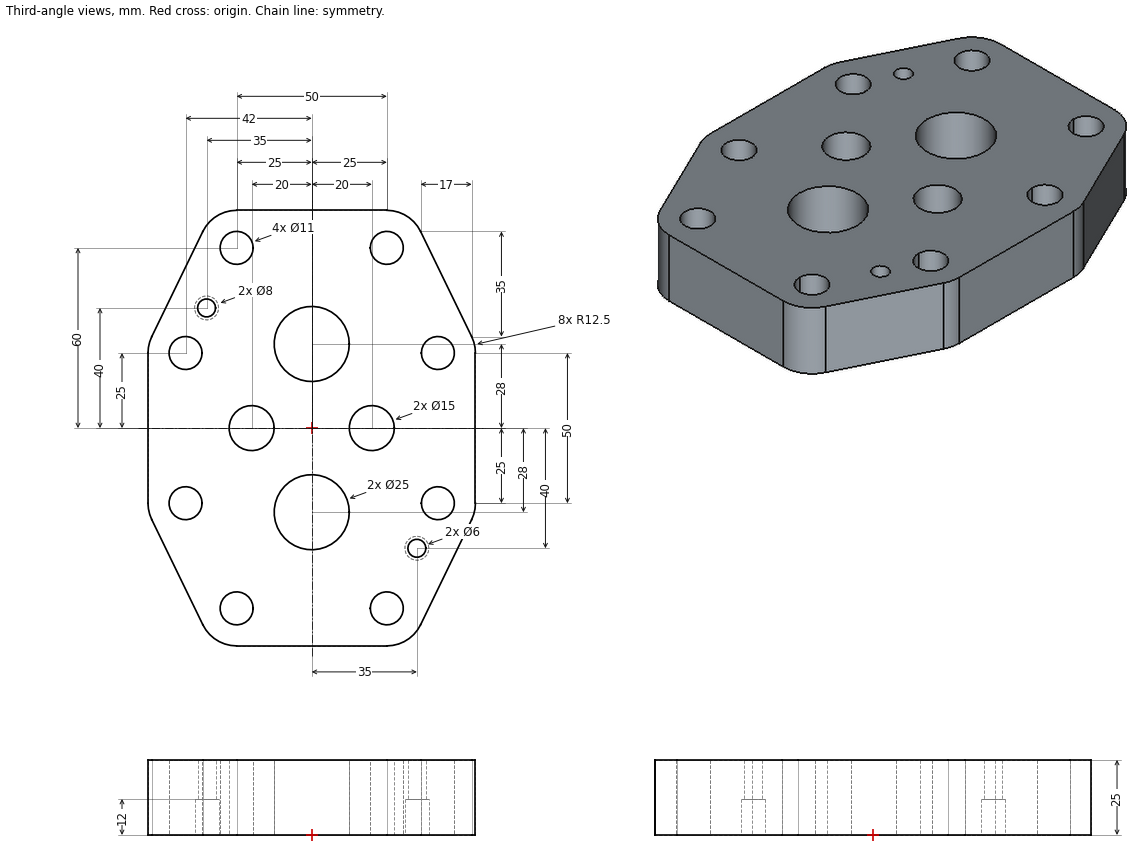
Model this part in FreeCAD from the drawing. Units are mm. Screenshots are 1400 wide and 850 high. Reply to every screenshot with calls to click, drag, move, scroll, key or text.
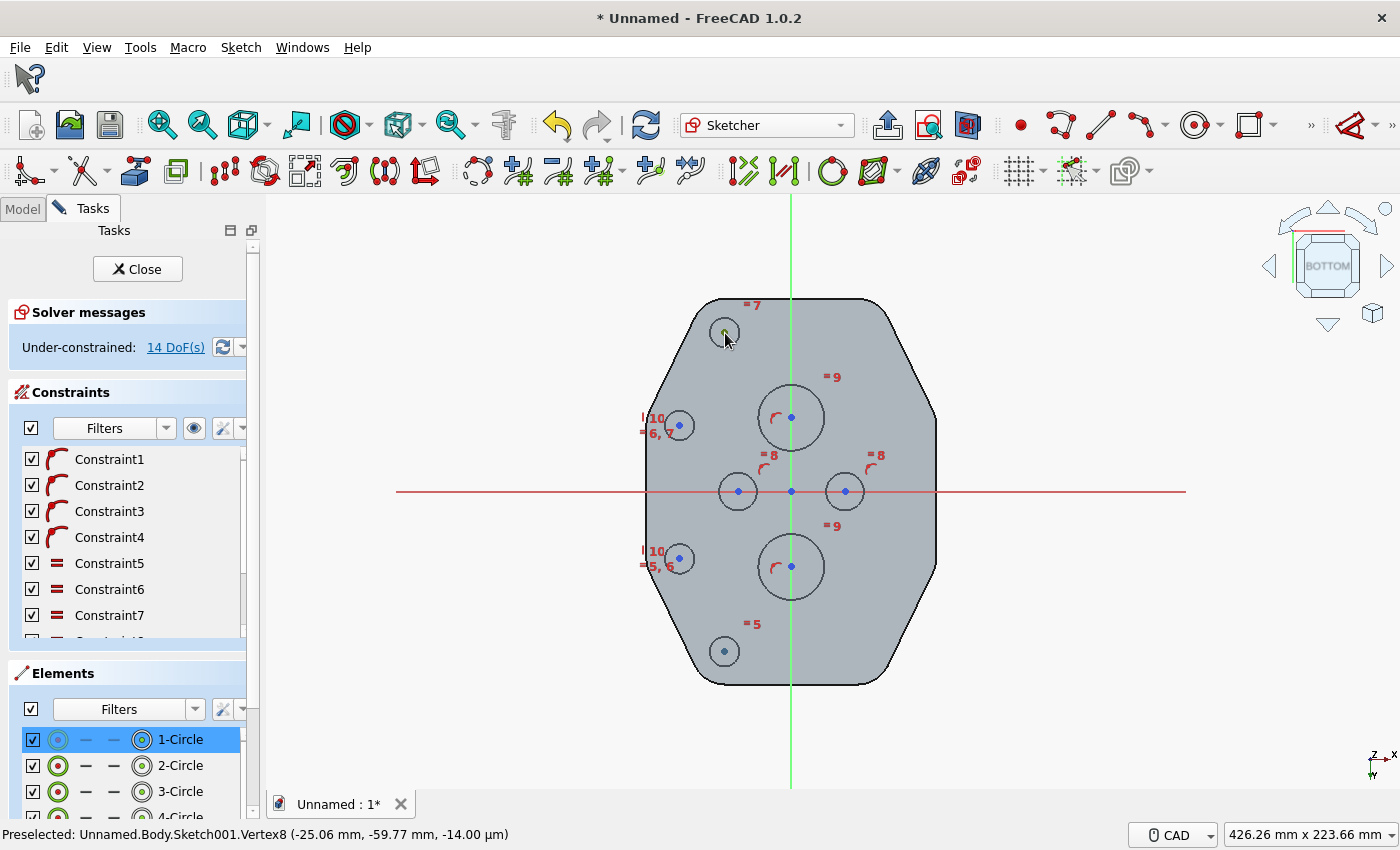
click(428, 492)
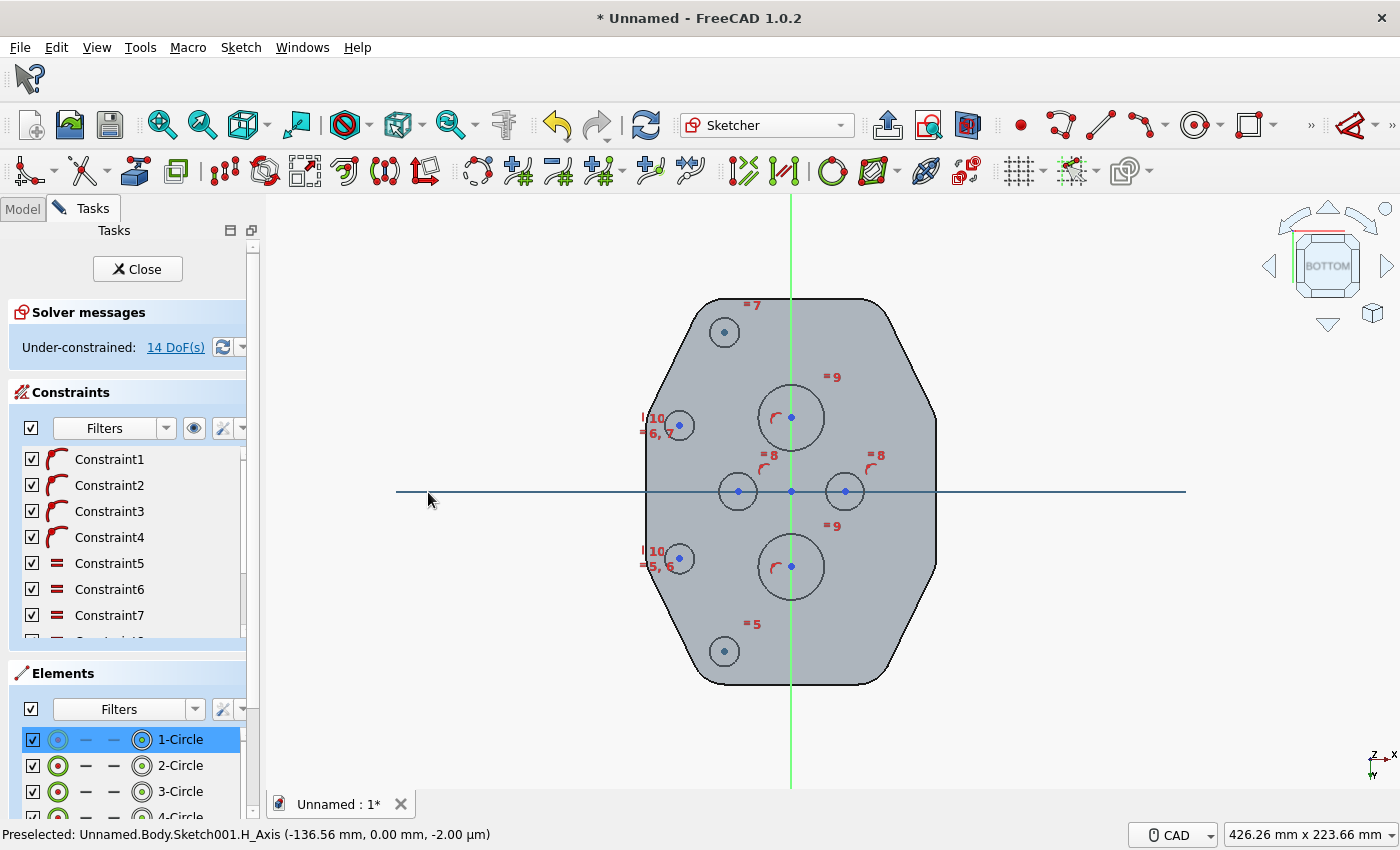
key(s)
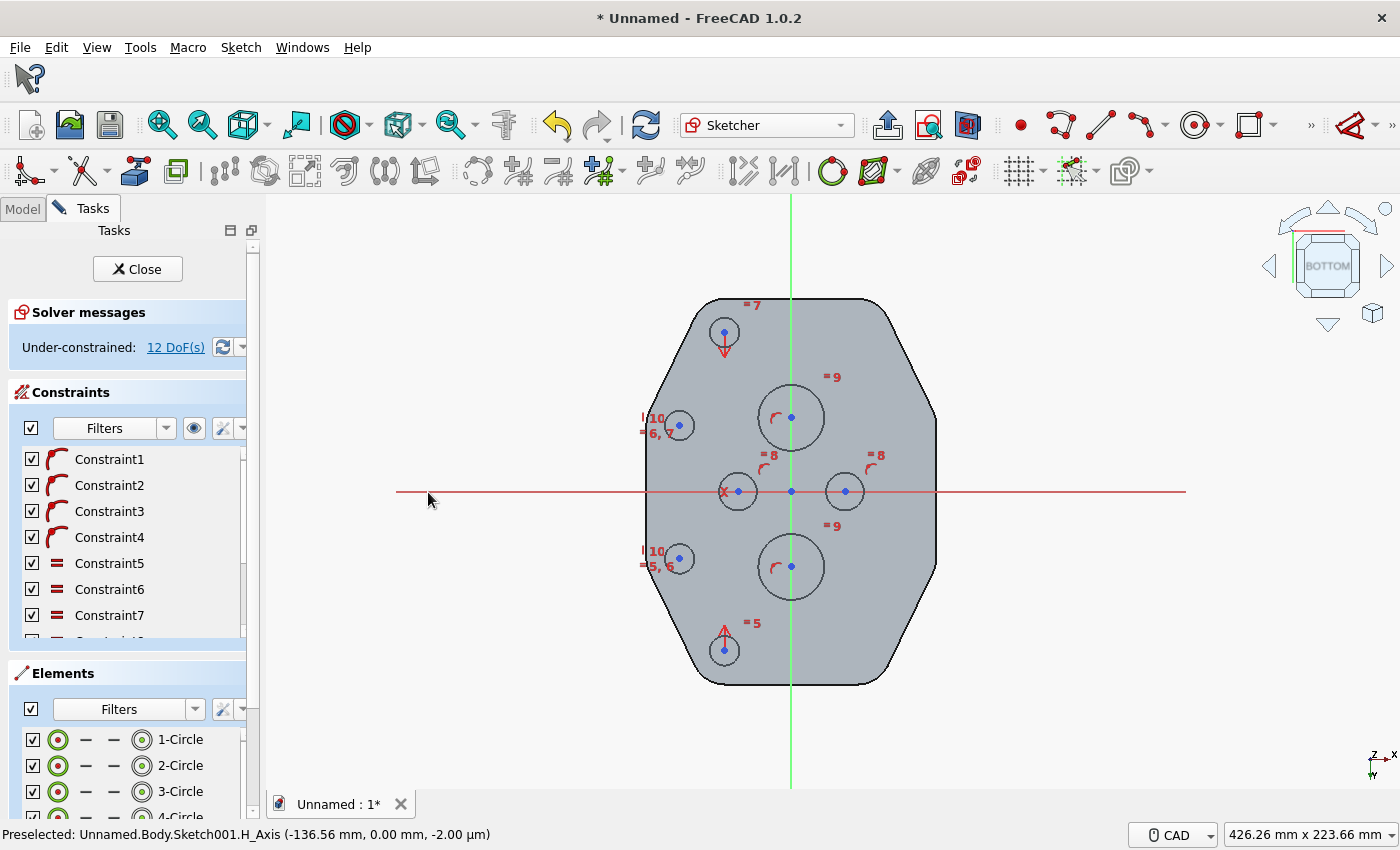
click(1350, 126)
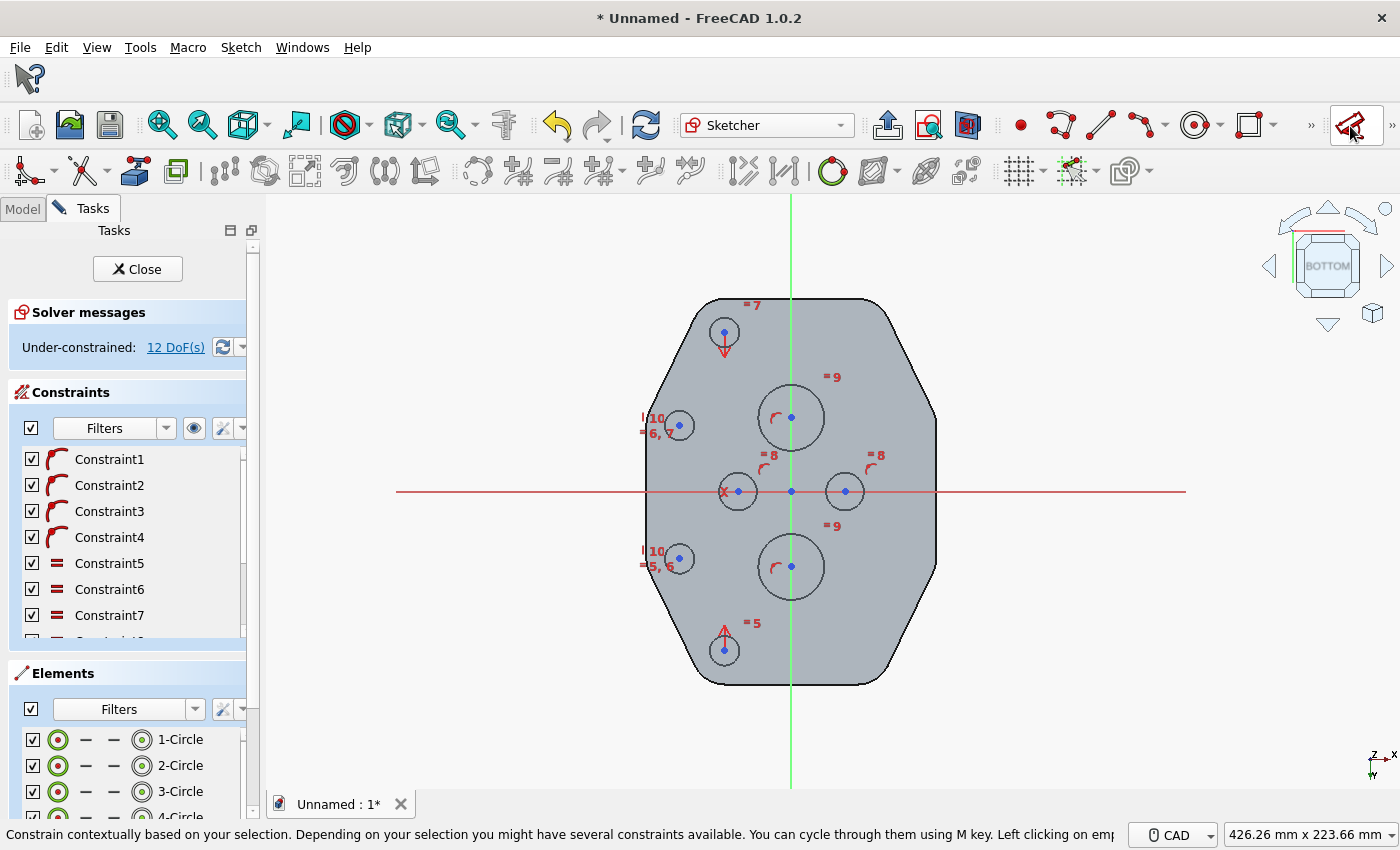
scroll(735, 640, up, 2)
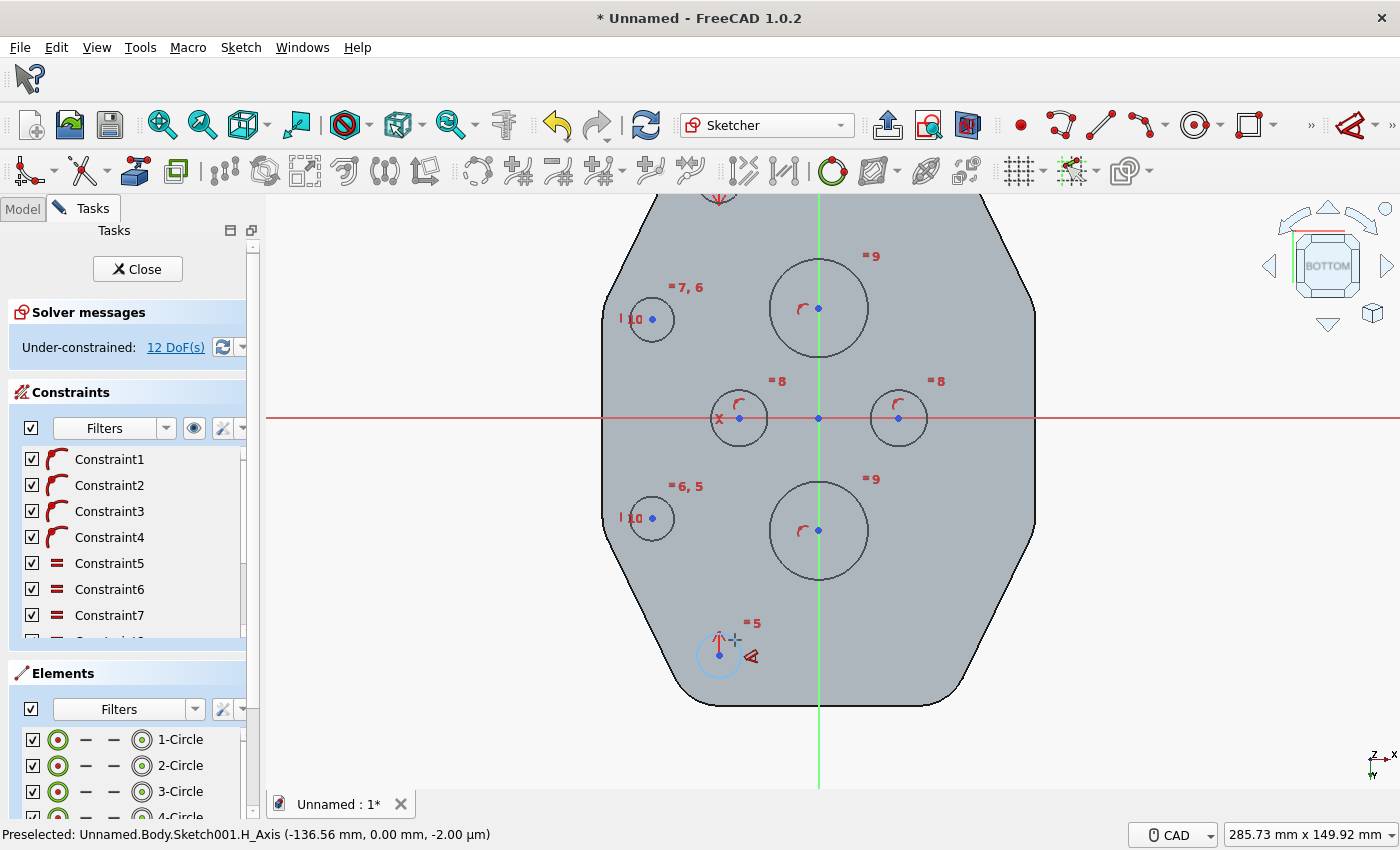
click(735, 640)
click(758, 617)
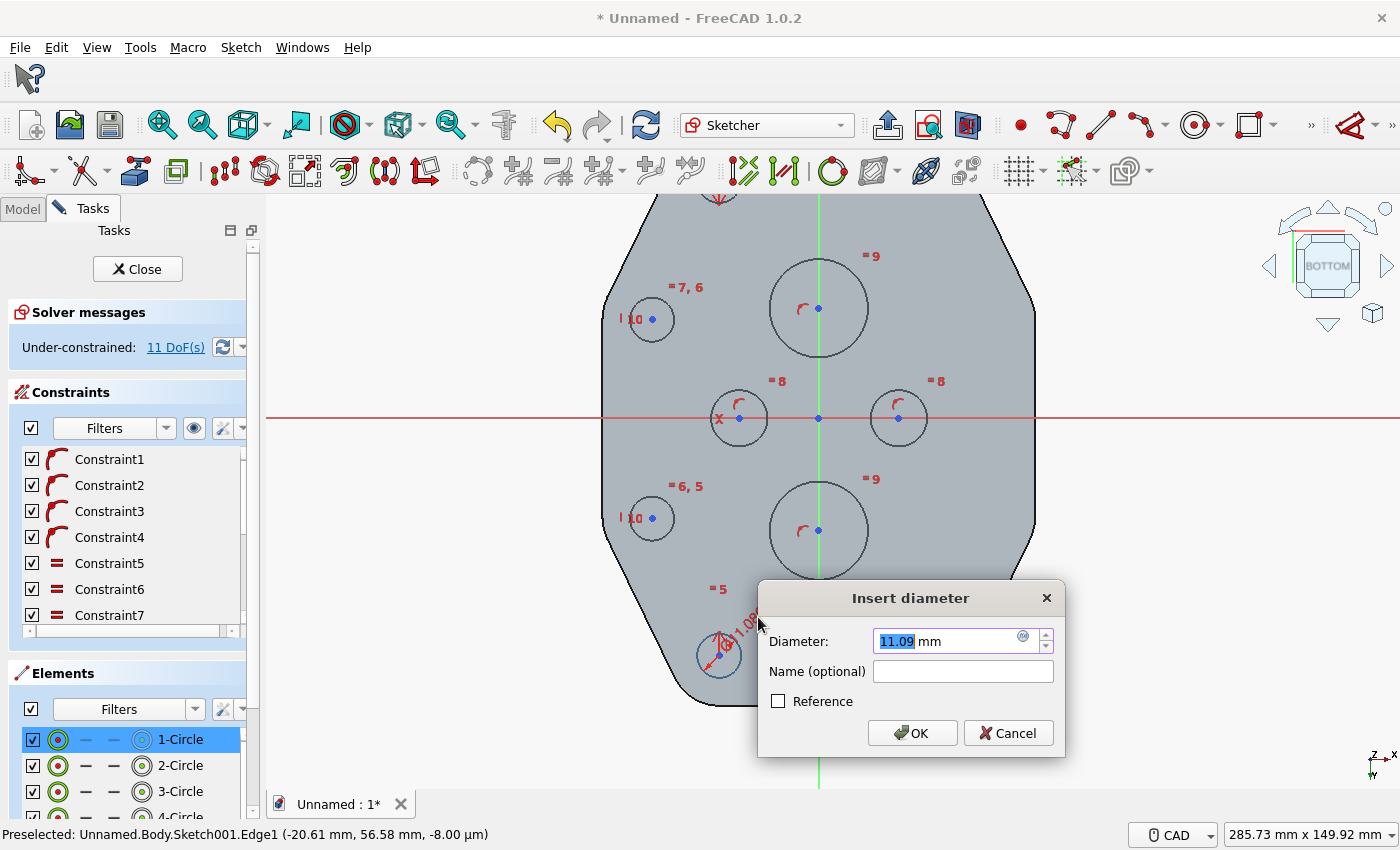
text(11)
key(Return)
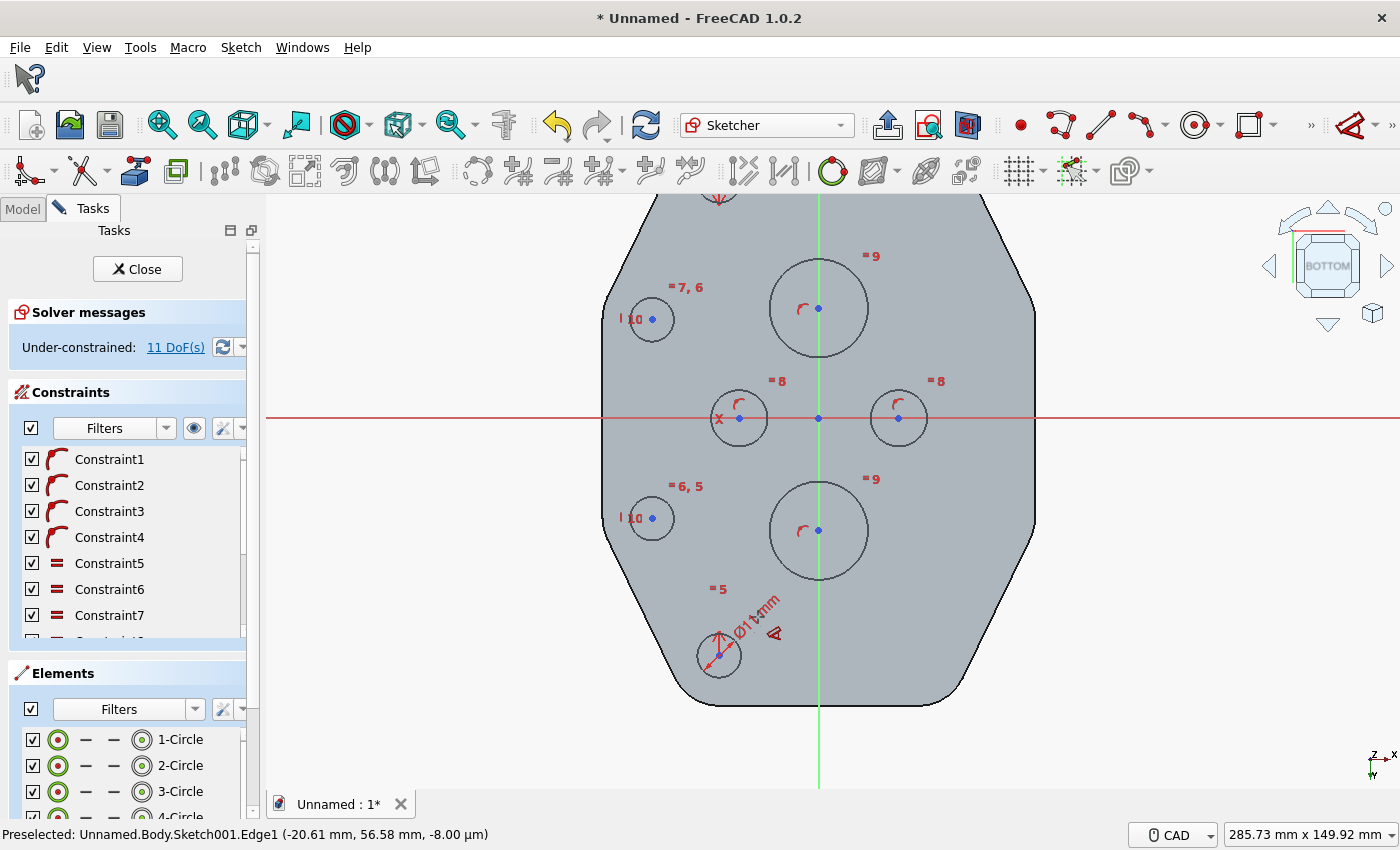
click(853, 273)
click(875, 250)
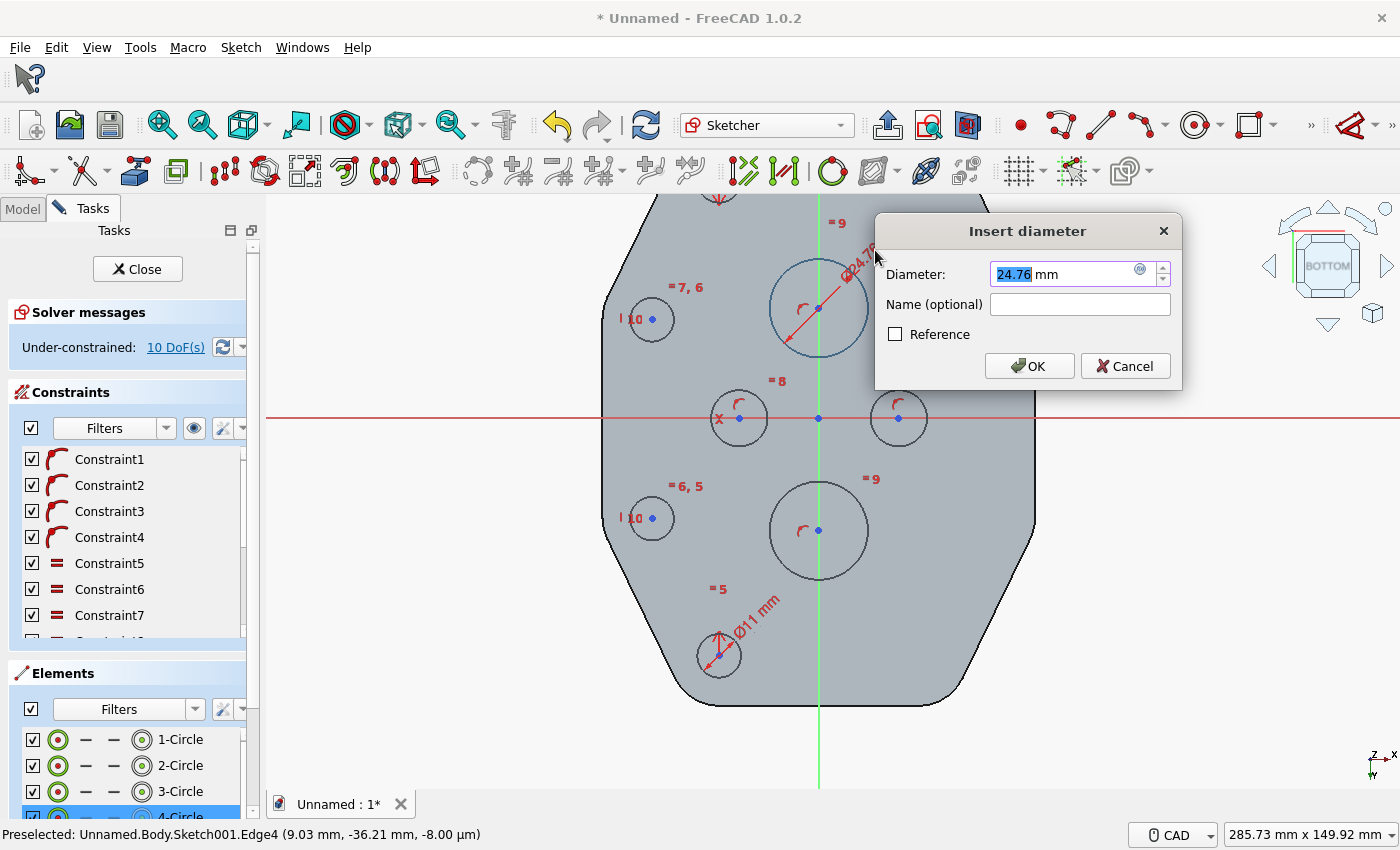
text(25)
key(Return)